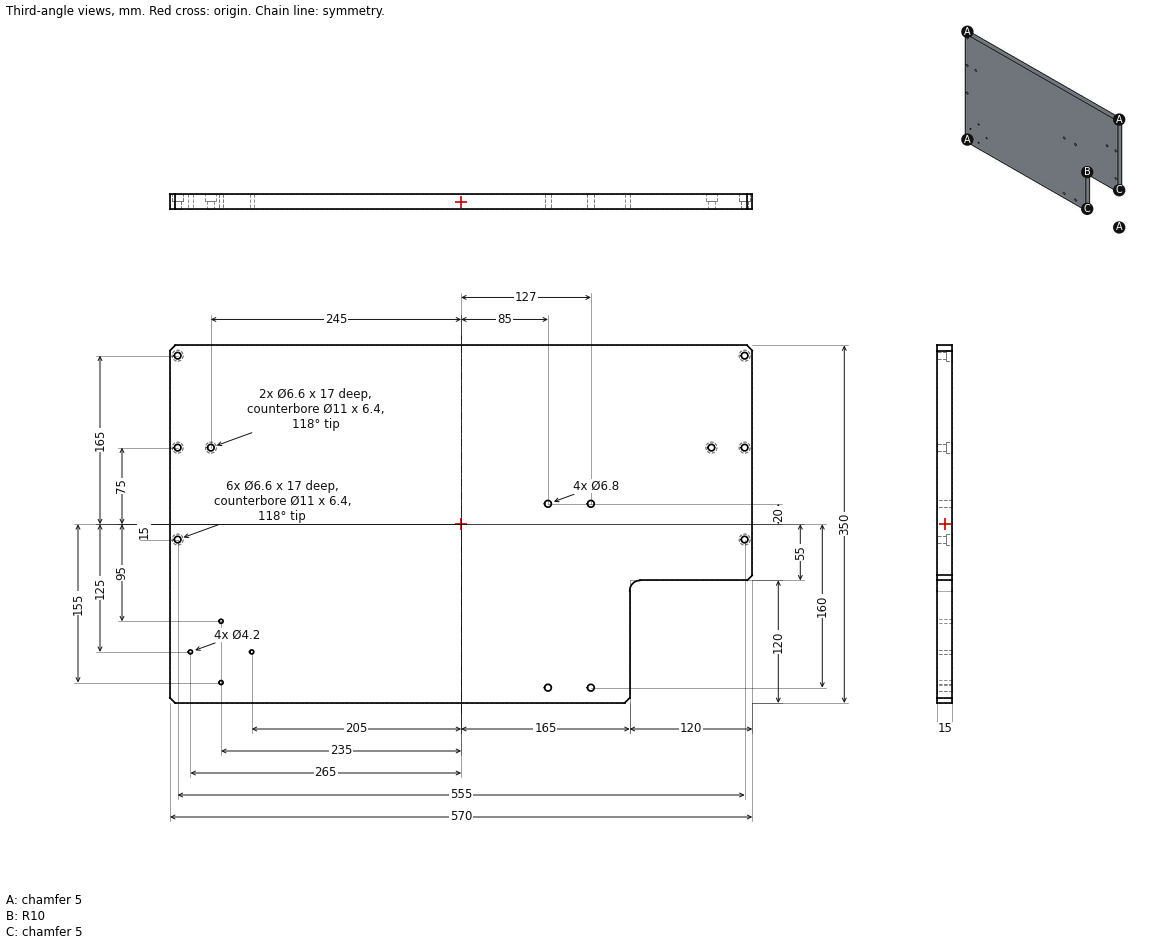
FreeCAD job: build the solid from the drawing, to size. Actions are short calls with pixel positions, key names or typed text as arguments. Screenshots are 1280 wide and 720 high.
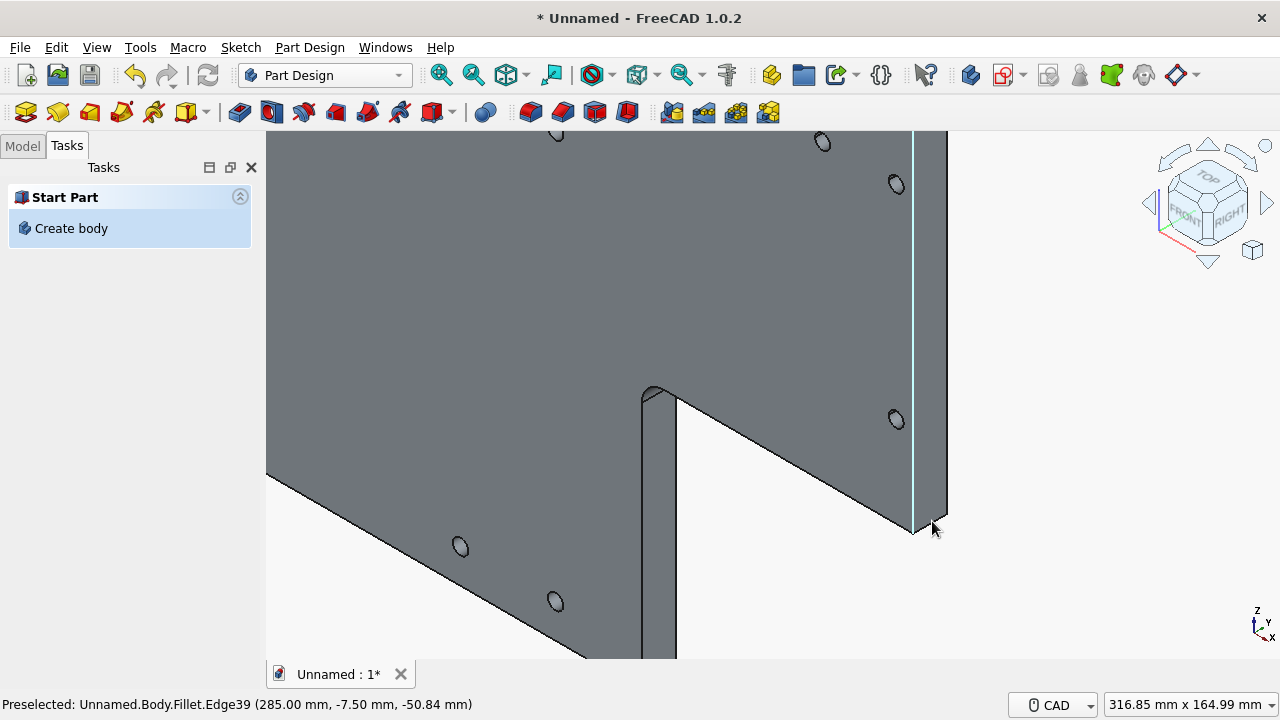
click(442, 76)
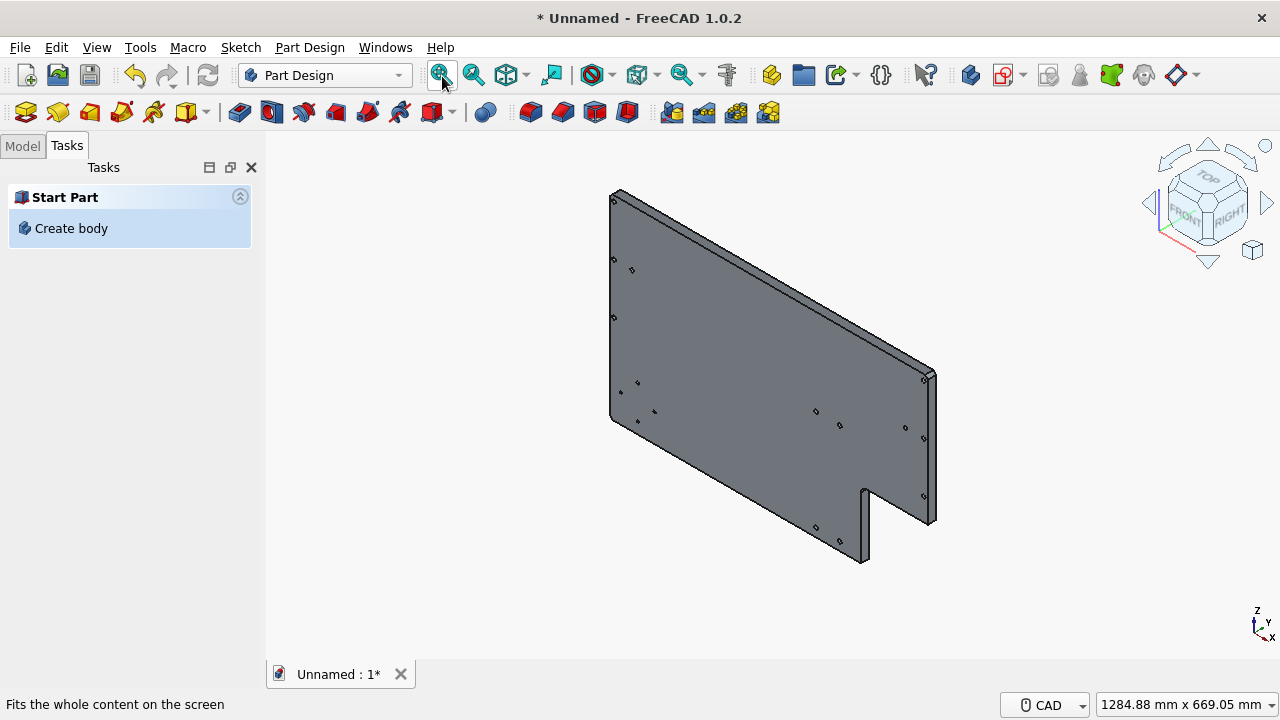
key(1)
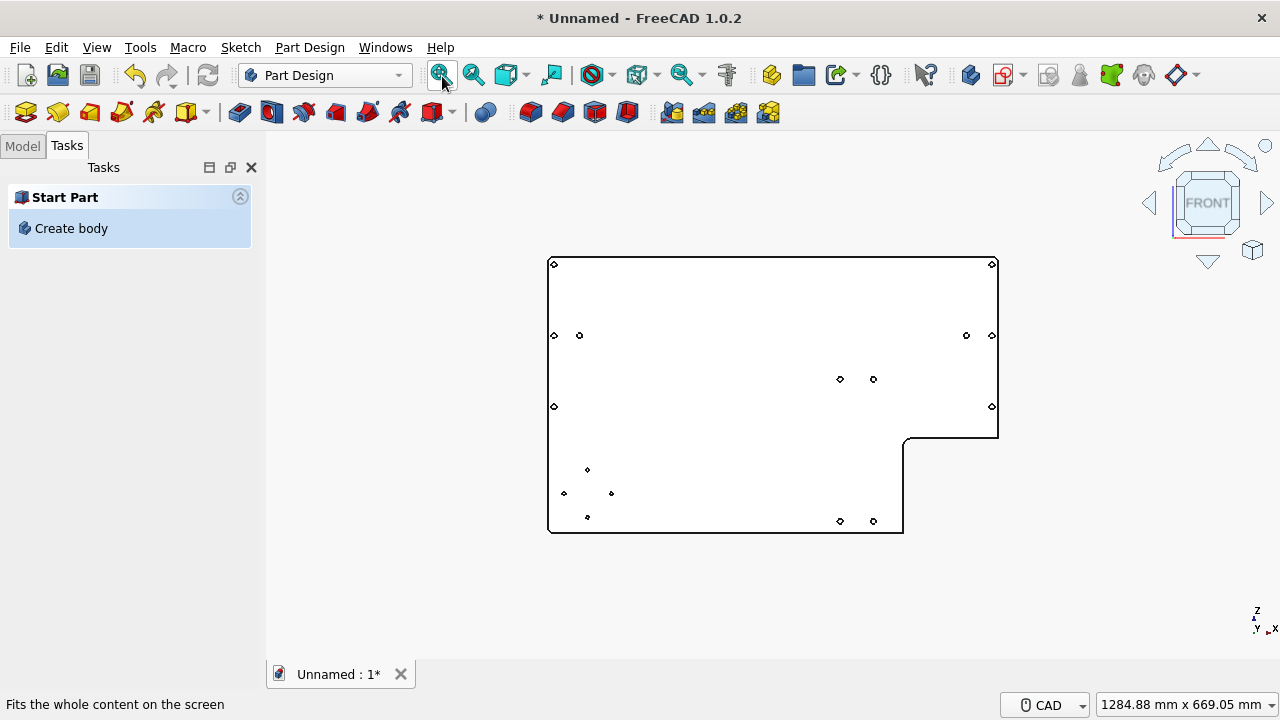
scroll(998, 437, up, 7)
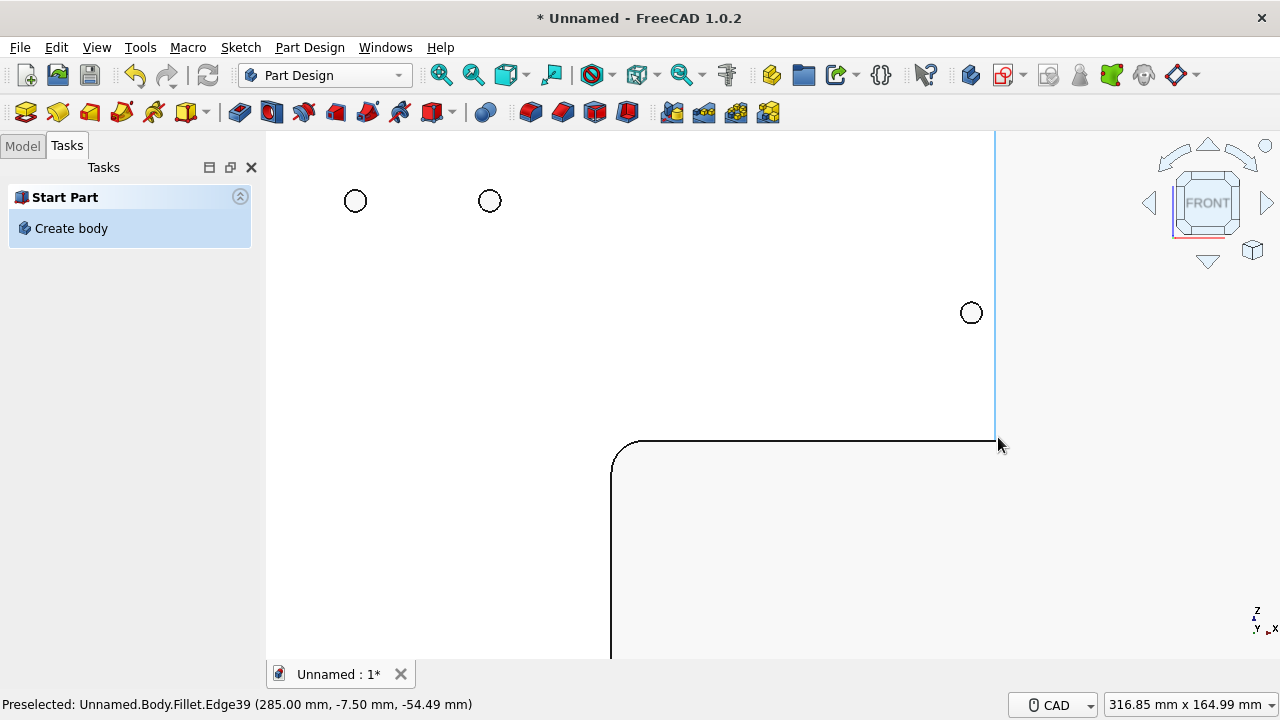
click(442, 76)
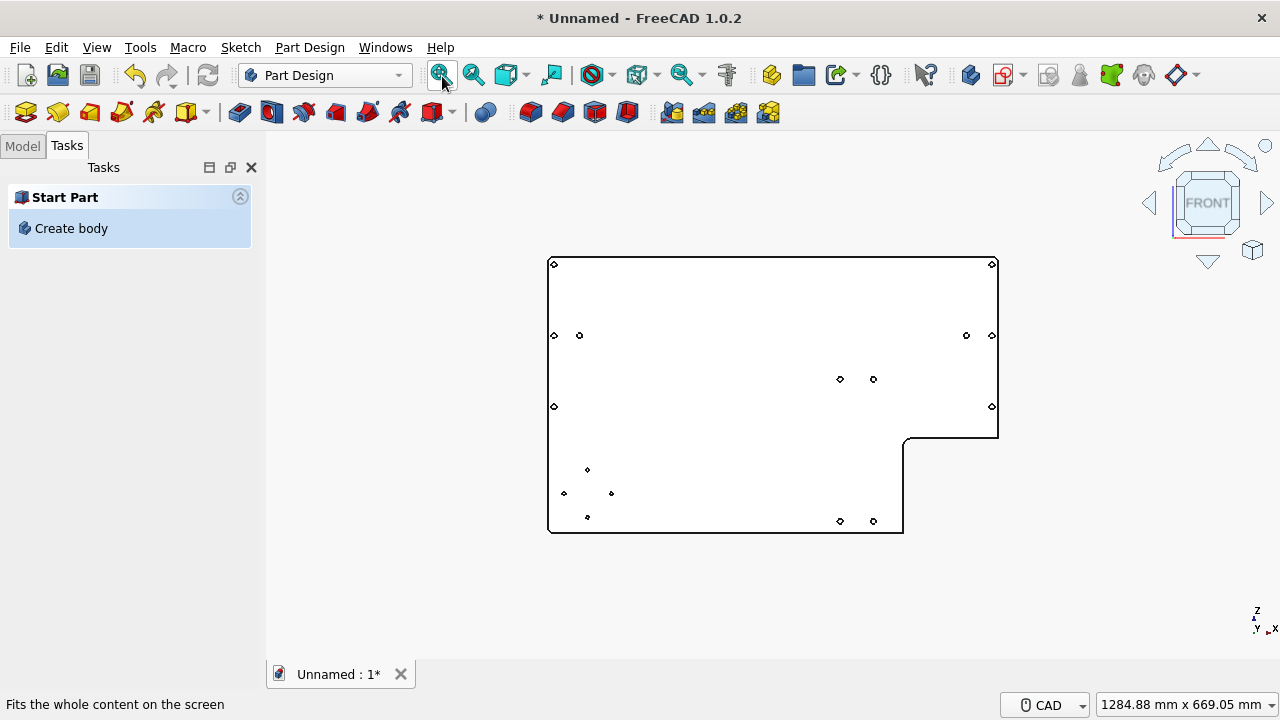
key(3)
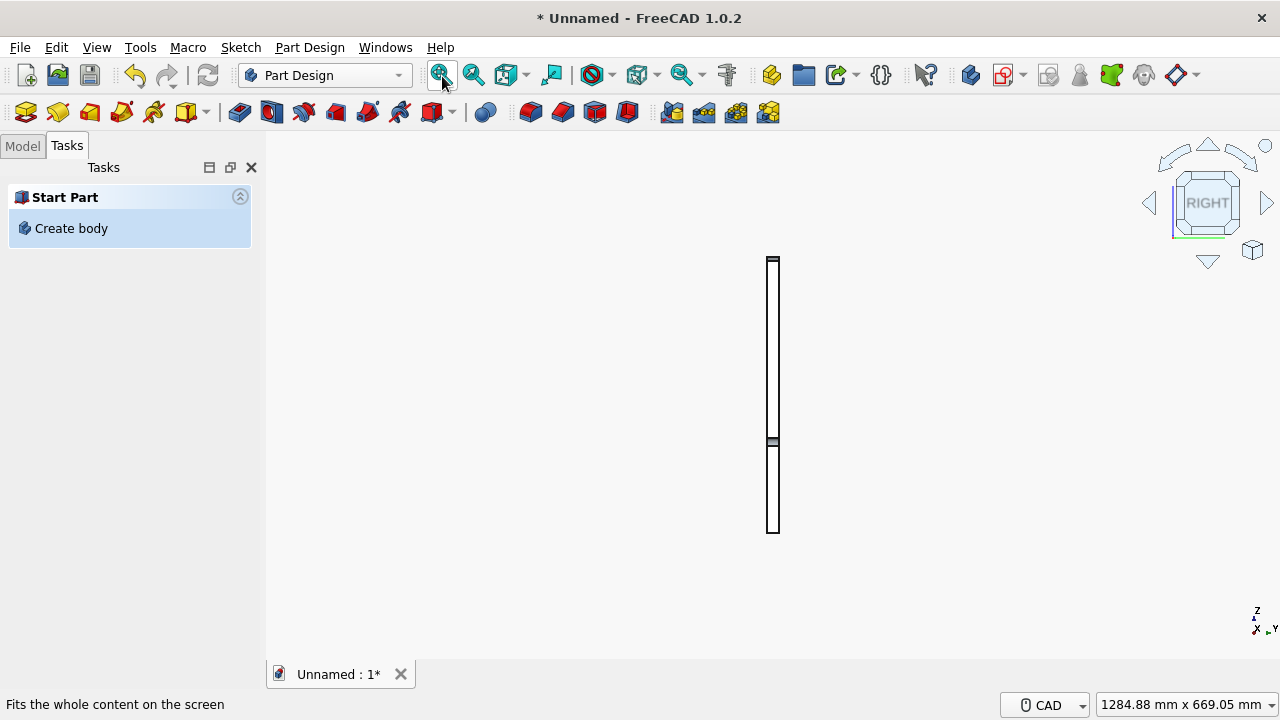
scroll(773, 437, up, 7)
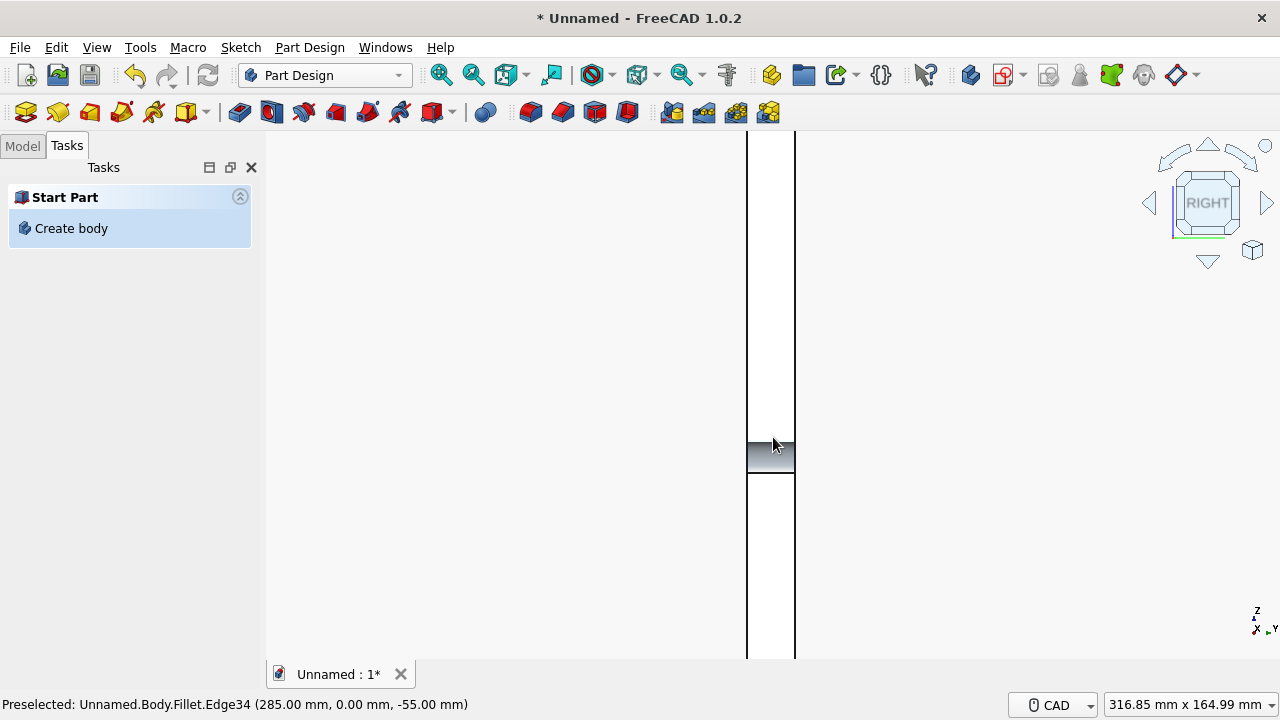
click(771, 440)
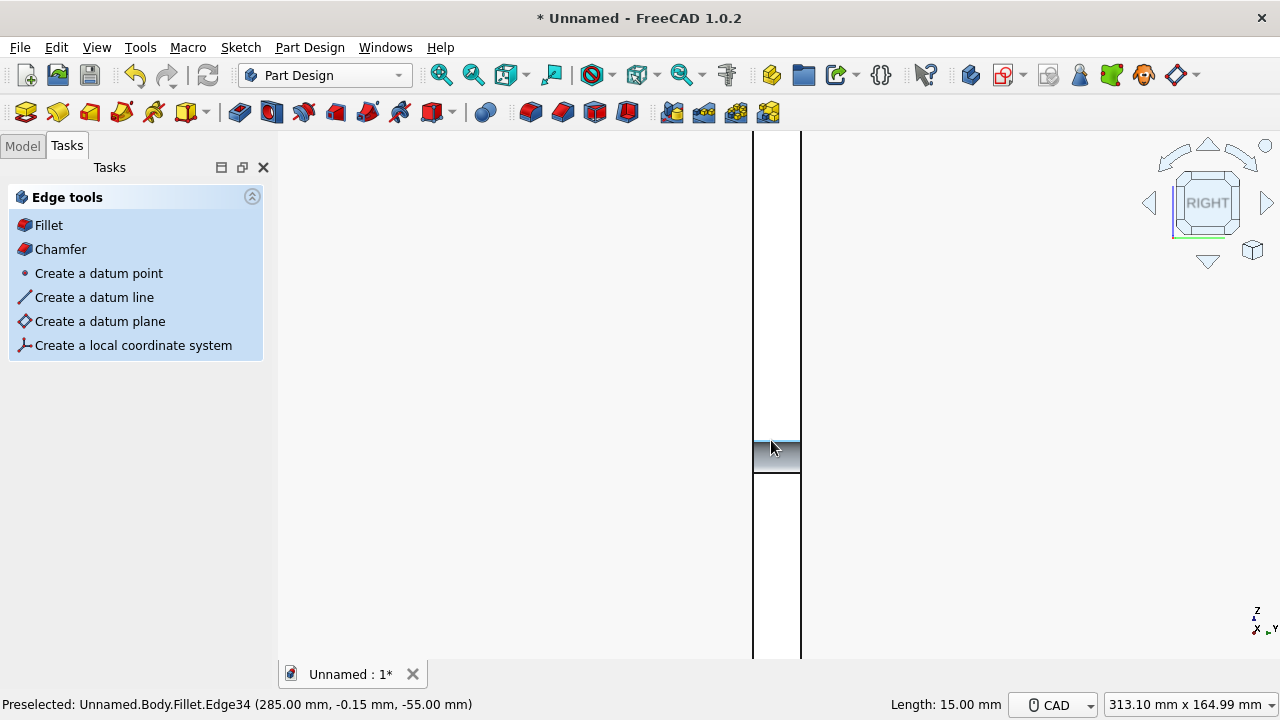
click(442, 76)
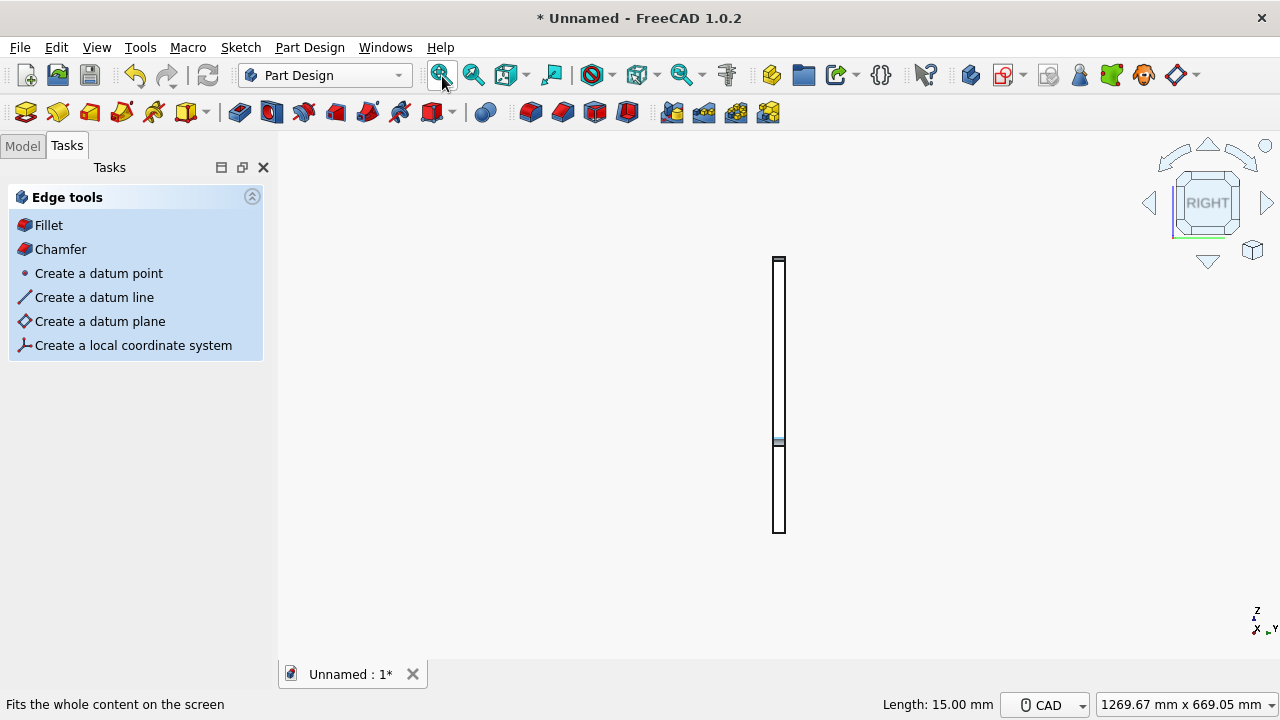
key(5)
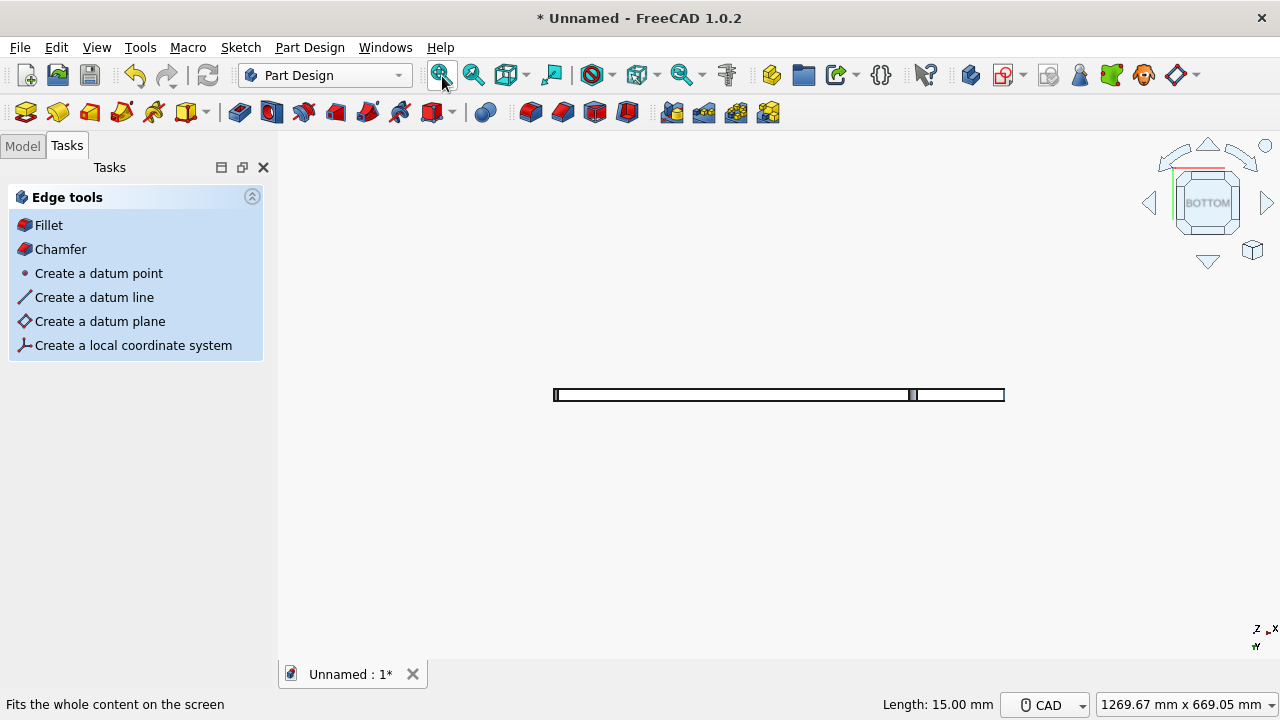
click(442, 76)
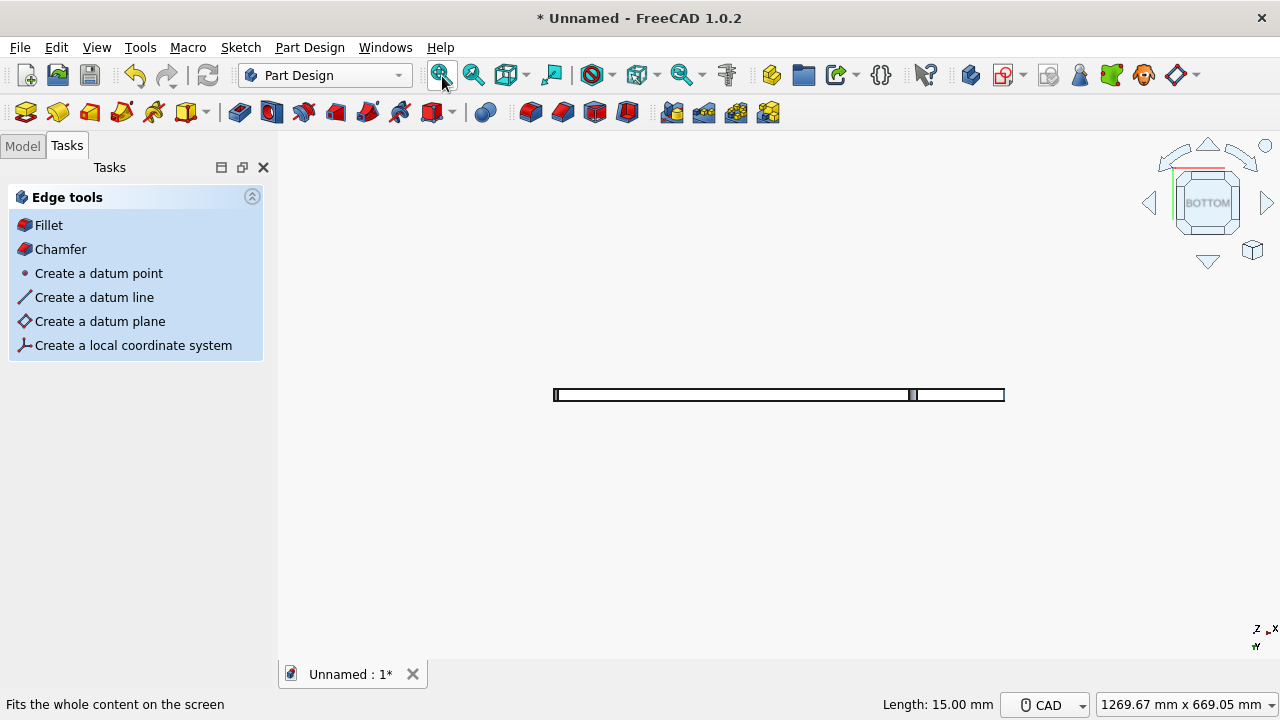
click(909, 395, ctrl)